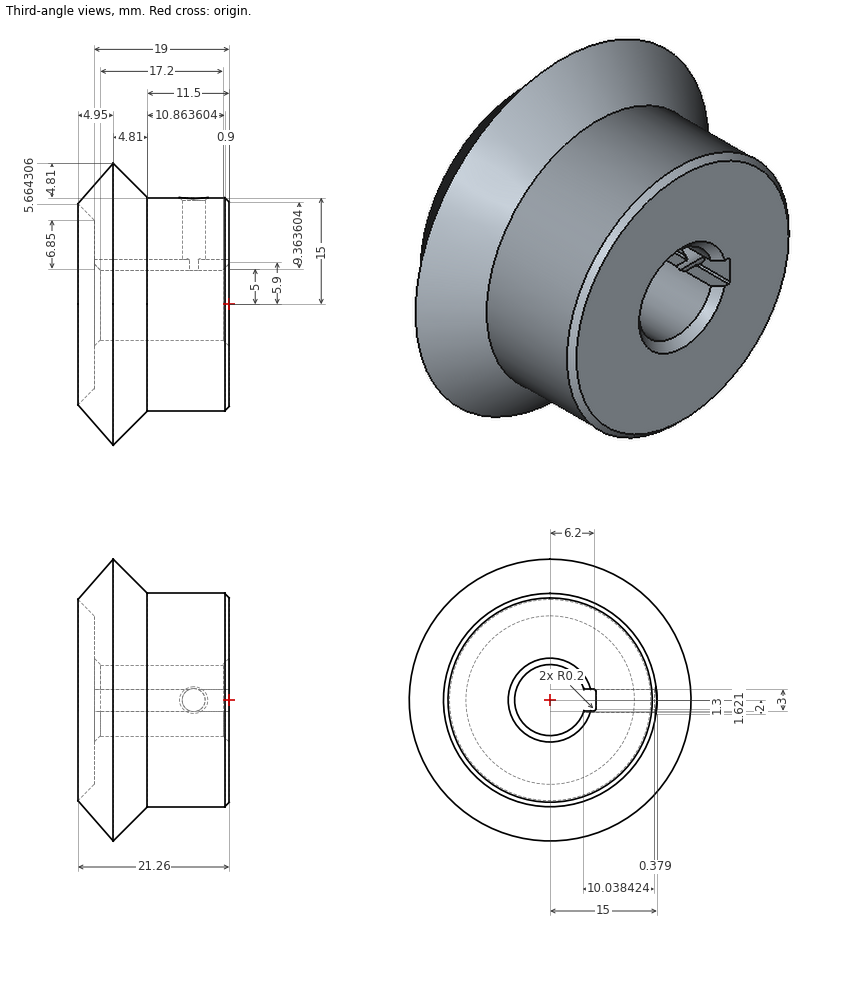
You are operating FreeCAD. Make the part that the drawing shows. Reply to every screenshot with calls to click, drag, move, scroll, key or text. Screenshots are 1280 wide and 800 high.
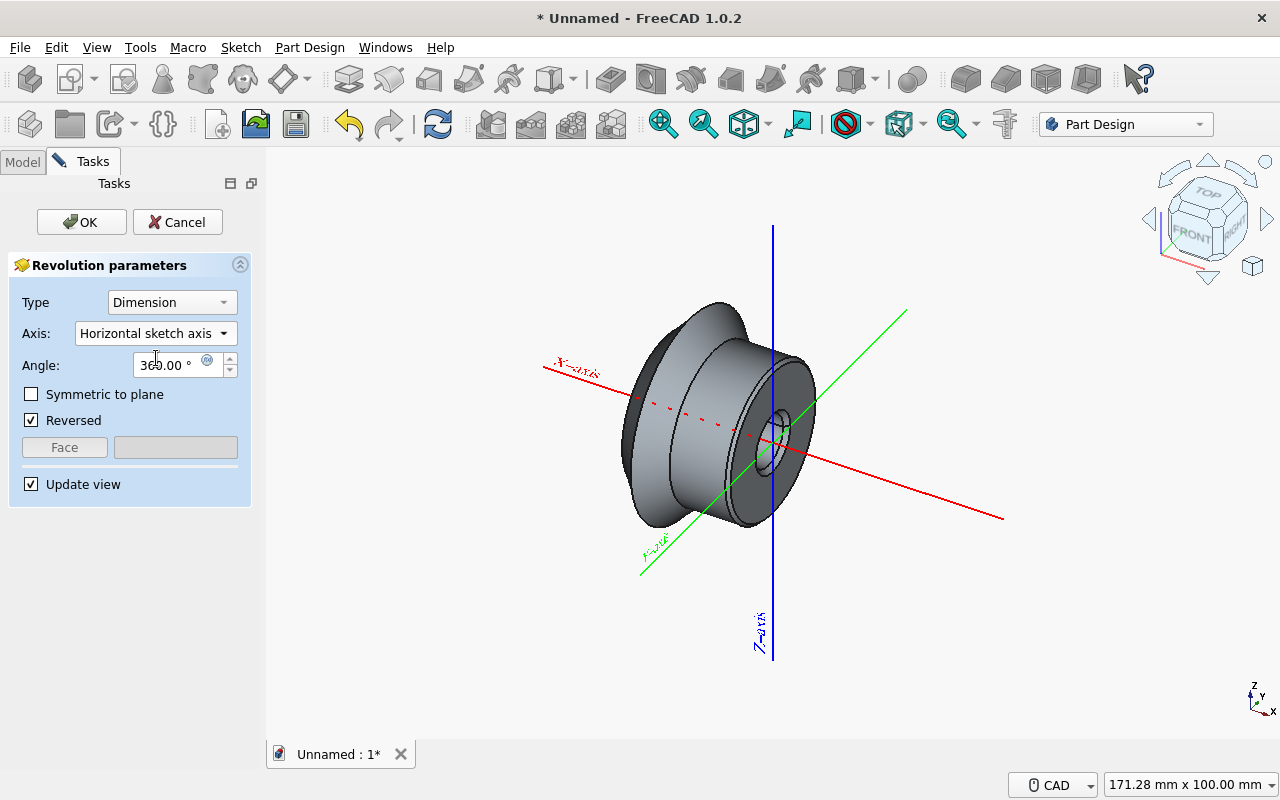
click(82, 222)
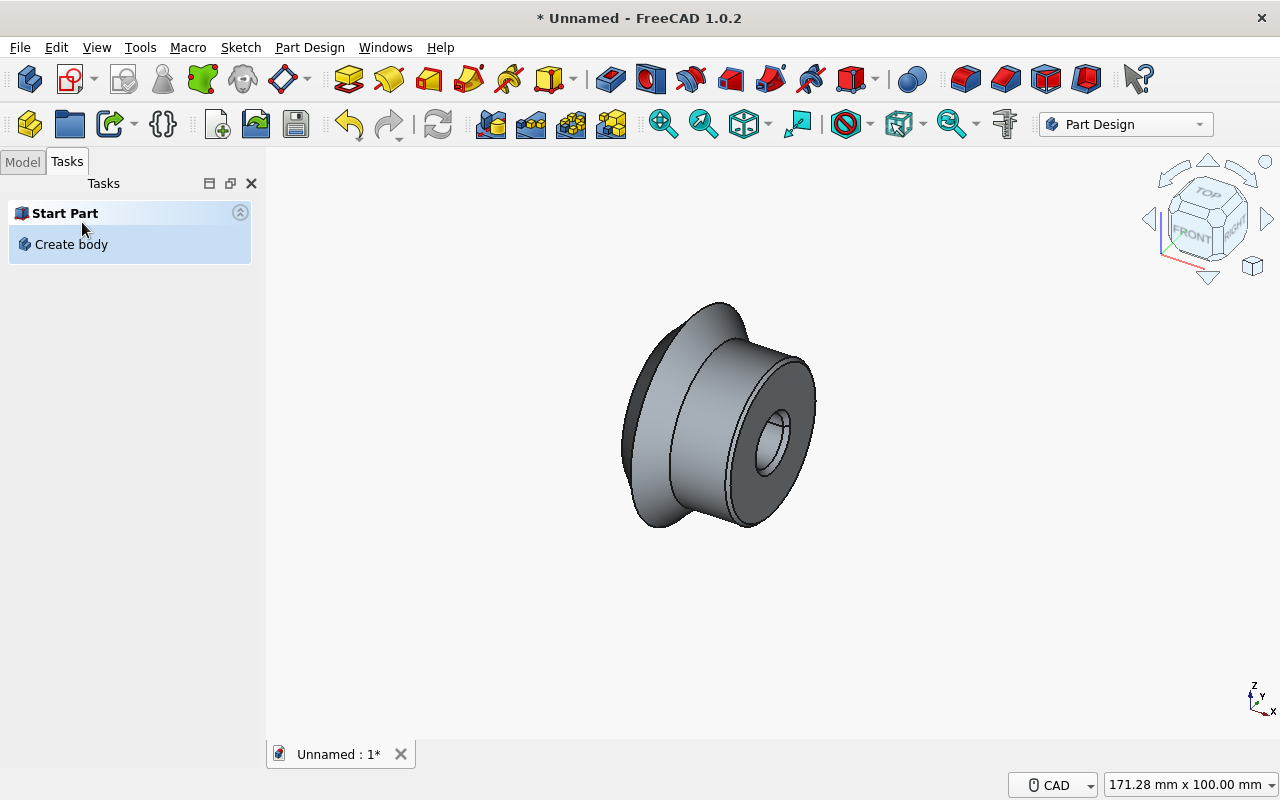
click(23, 161)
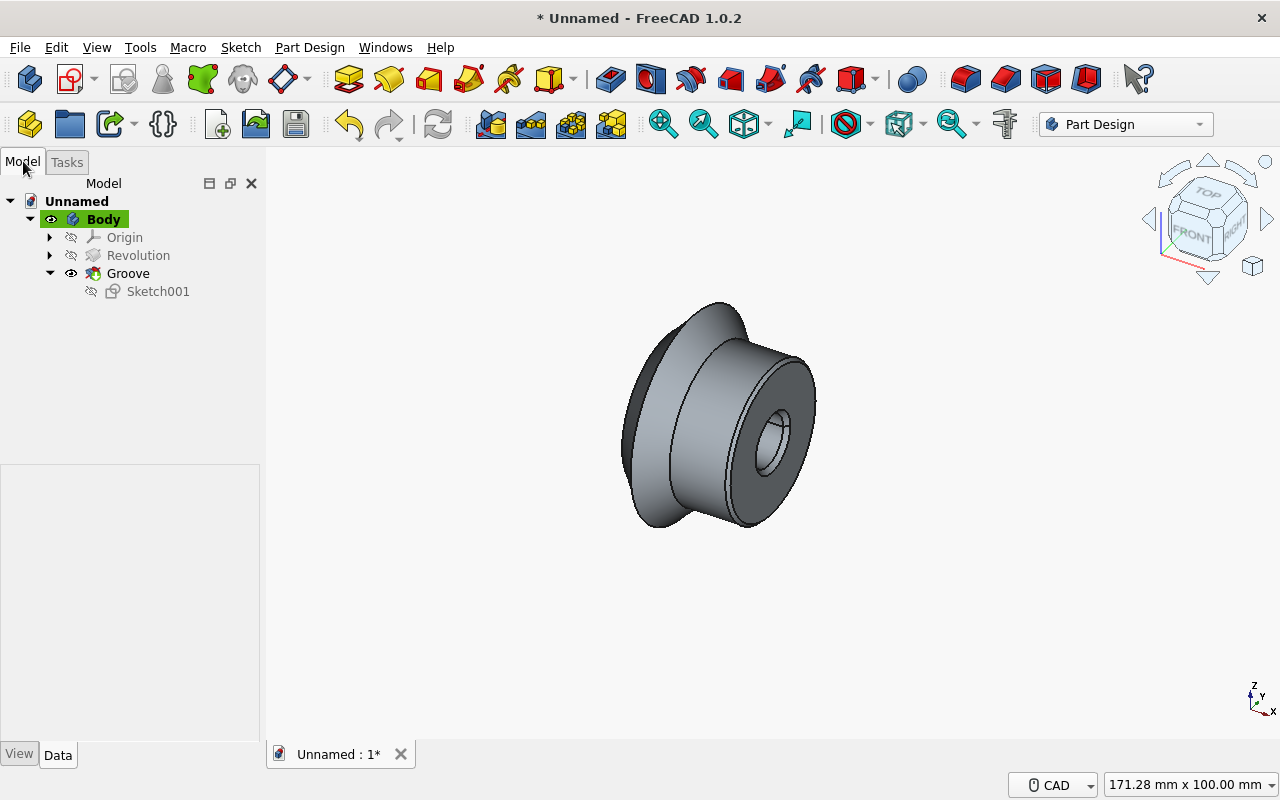
click(50, 237)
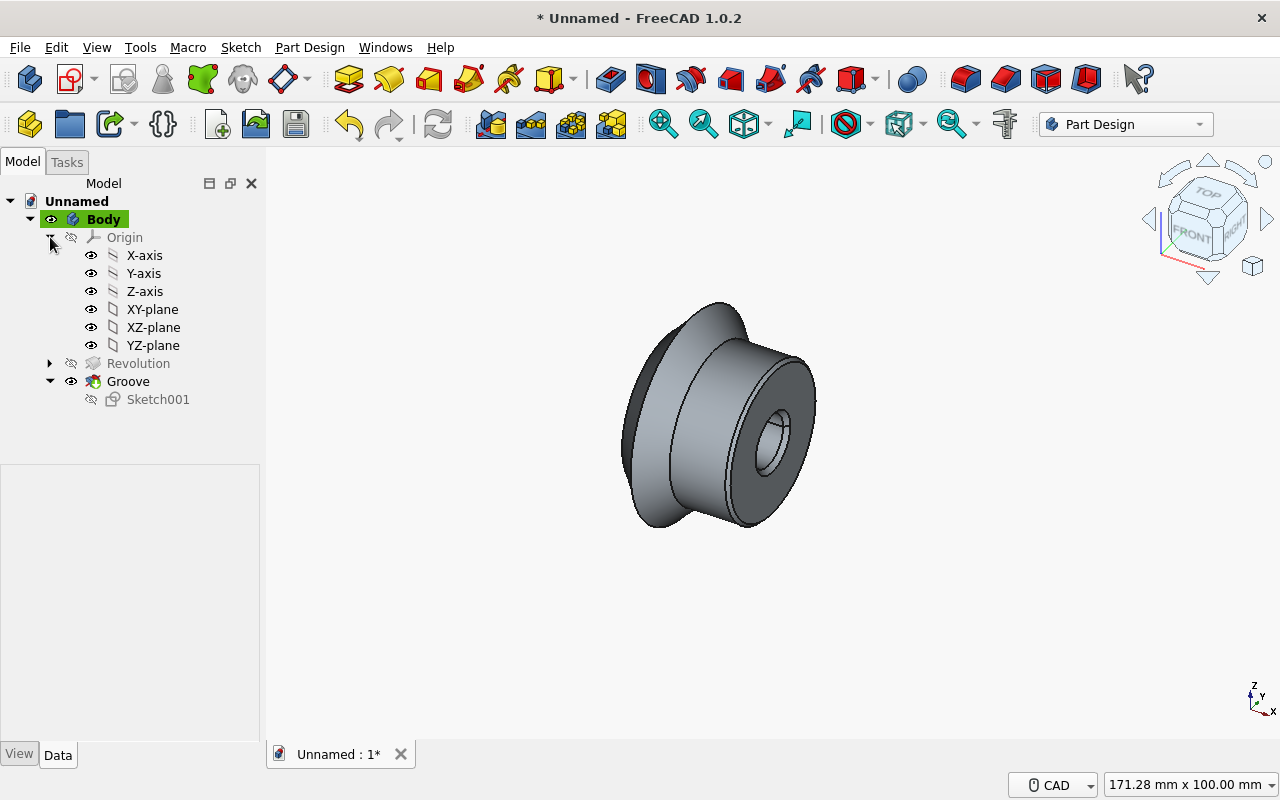
click(136, 345)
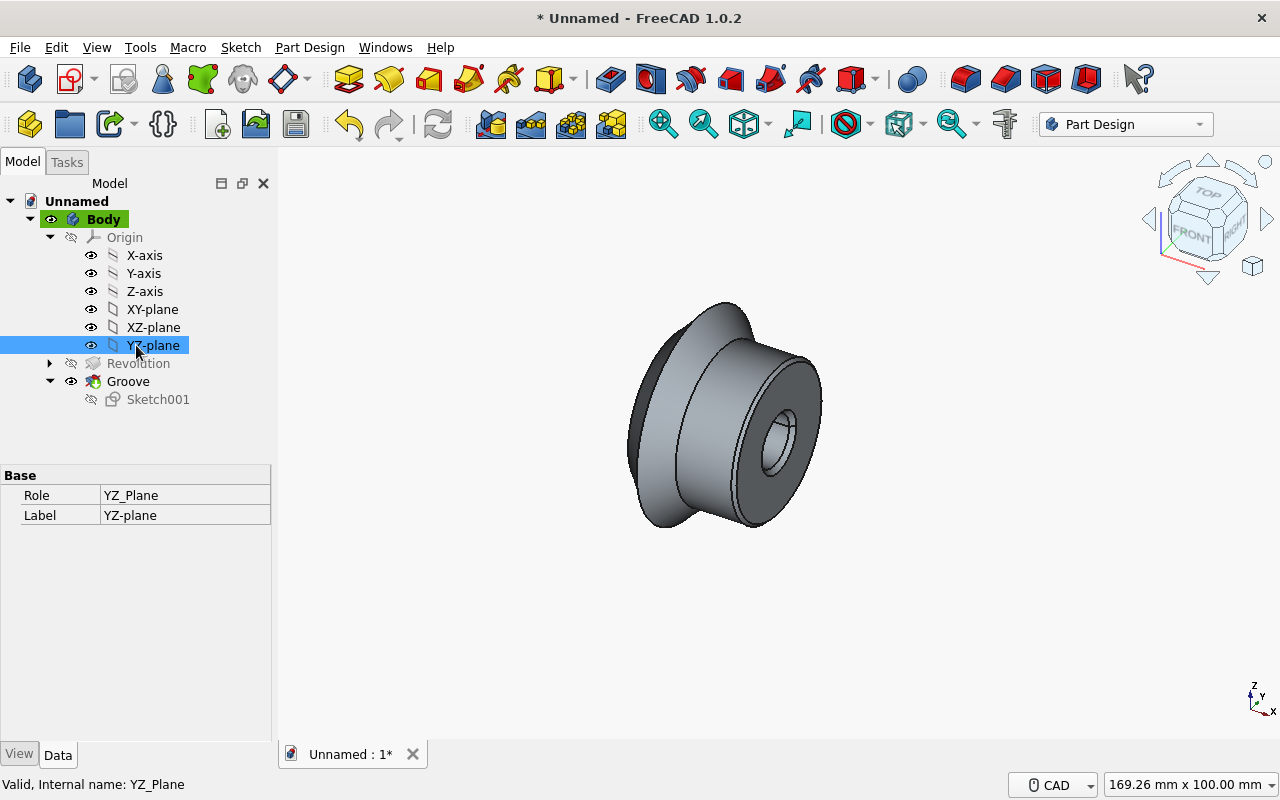
click(284, 80)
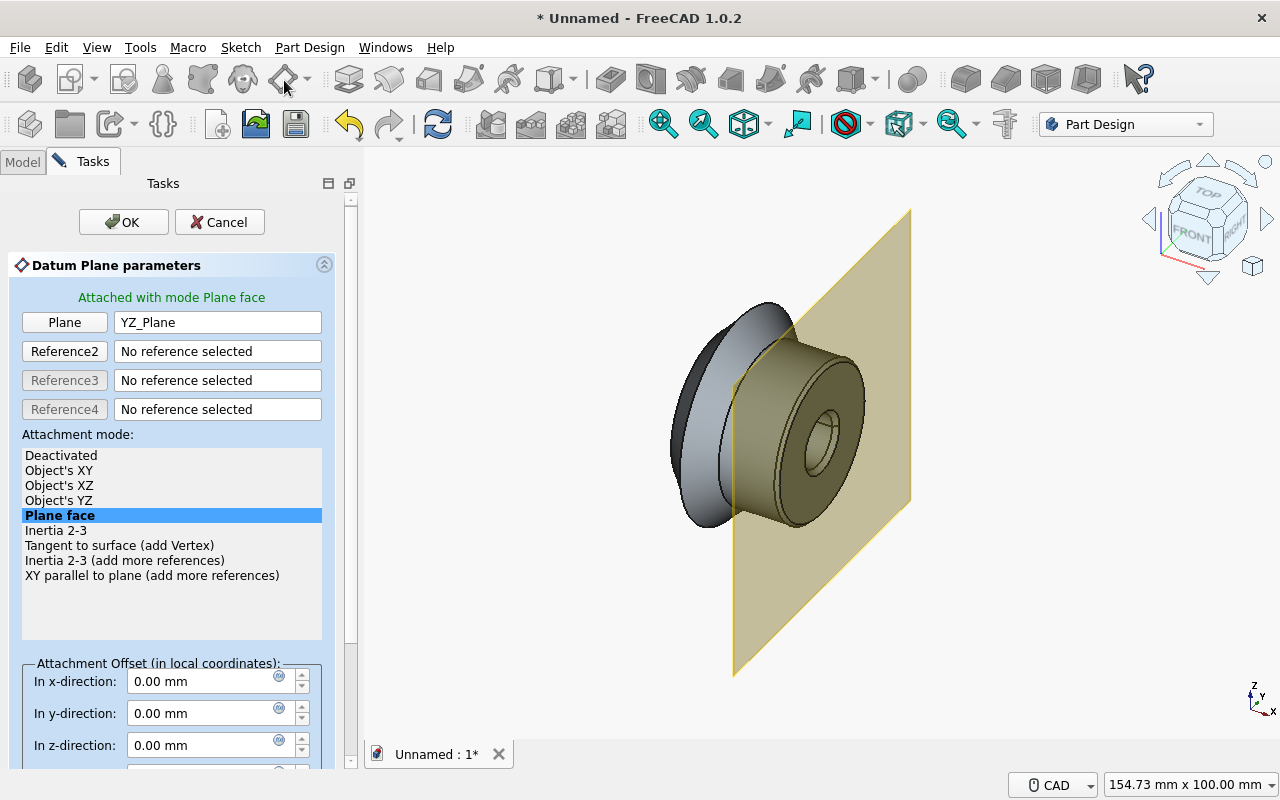
triple_click(210, 745)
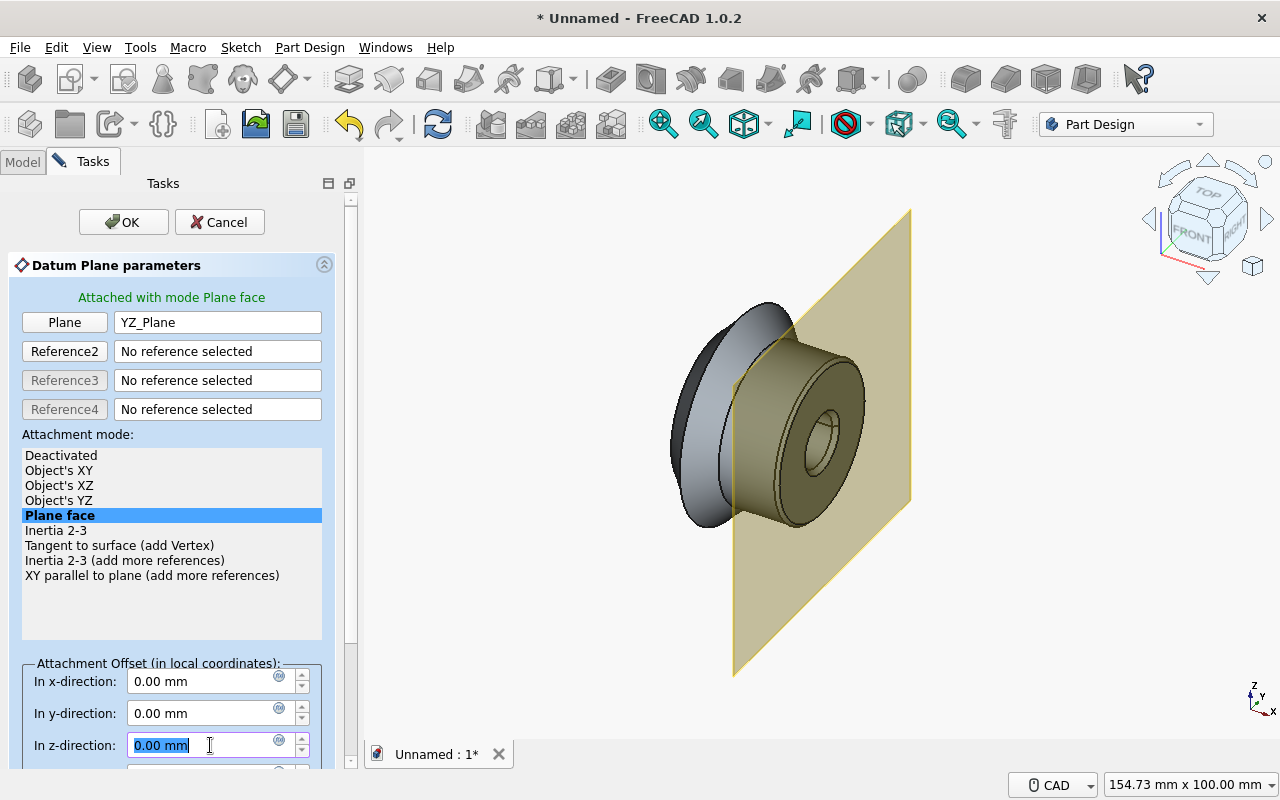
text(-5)
key(Tab)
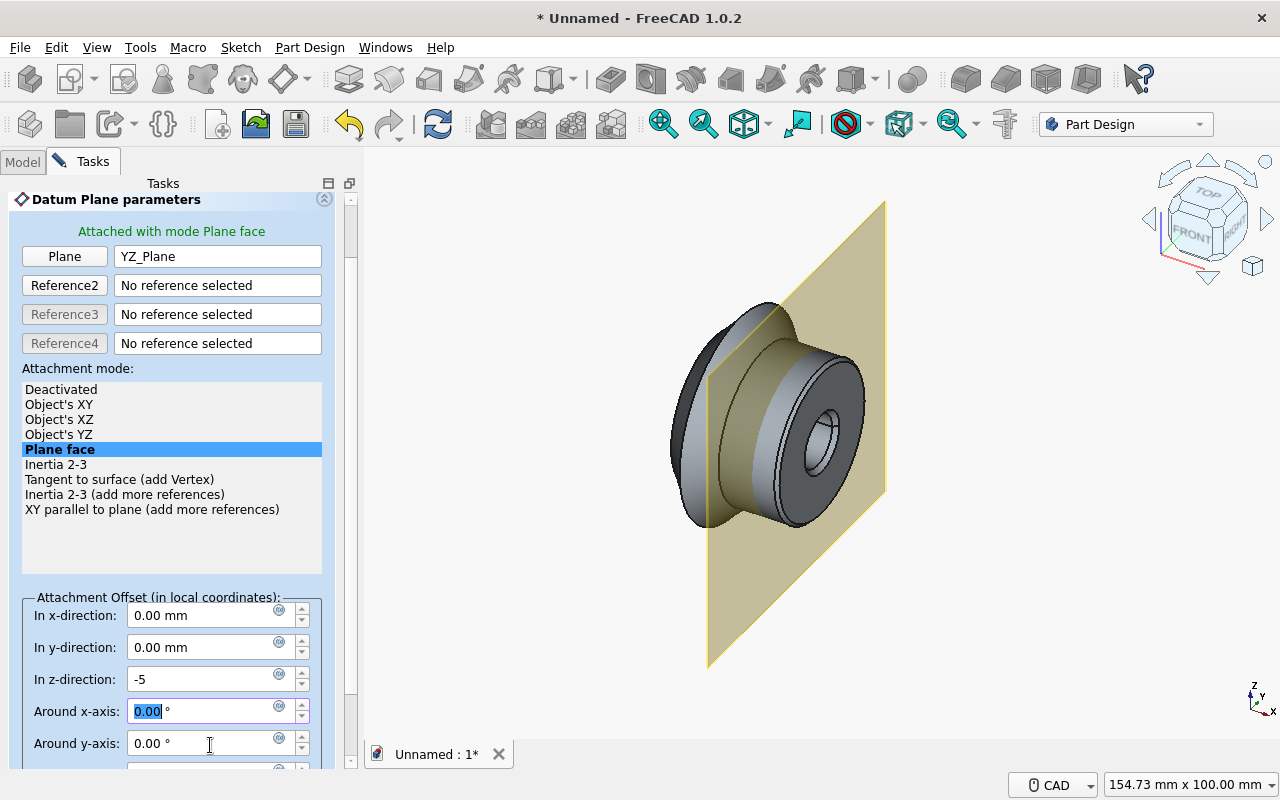
scroll(351, 480, up, 2)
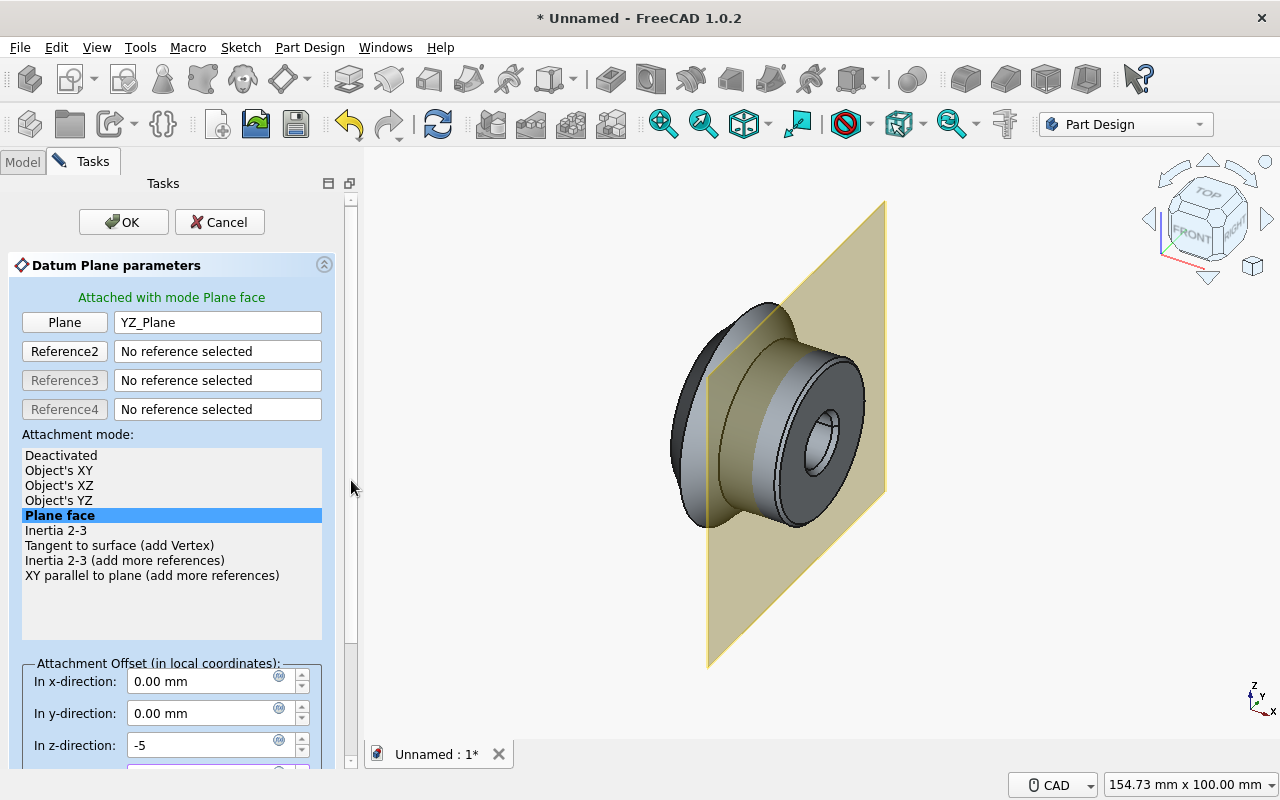
click(124, 222)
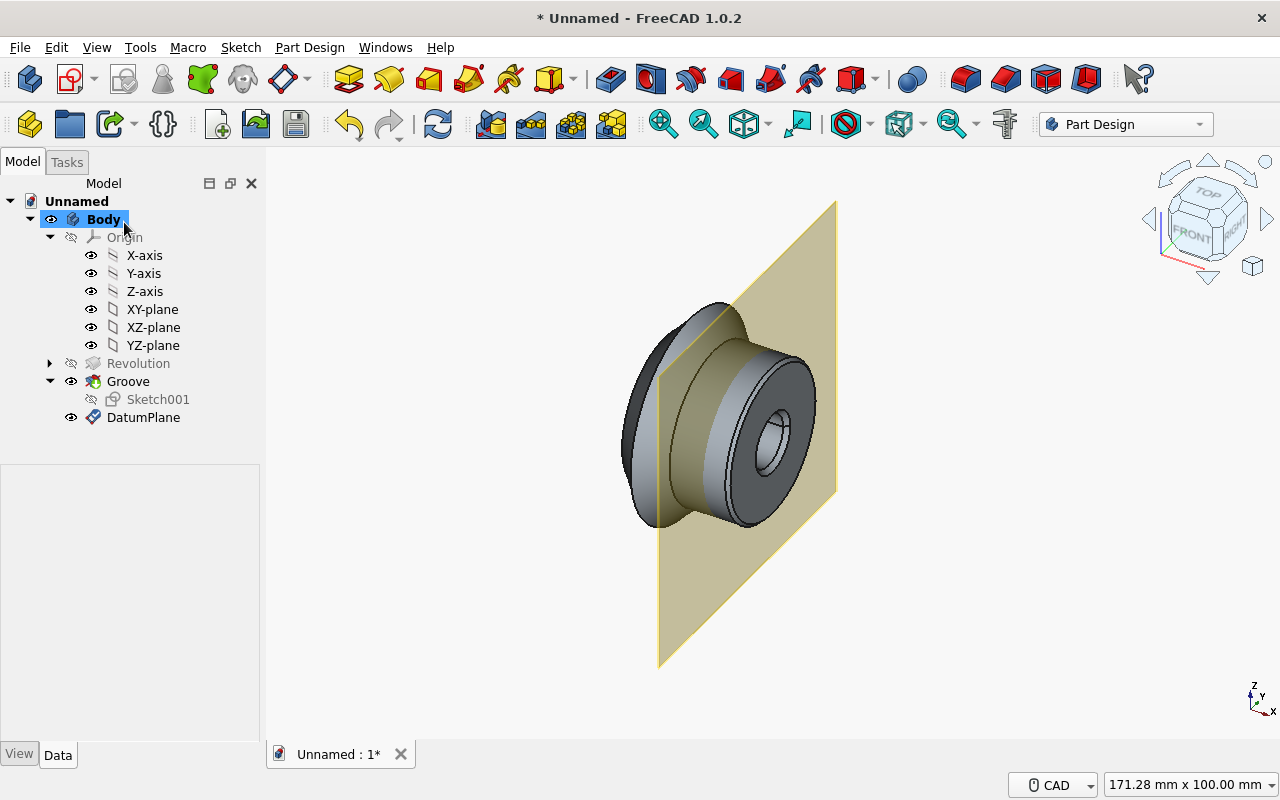
click(116, 417)